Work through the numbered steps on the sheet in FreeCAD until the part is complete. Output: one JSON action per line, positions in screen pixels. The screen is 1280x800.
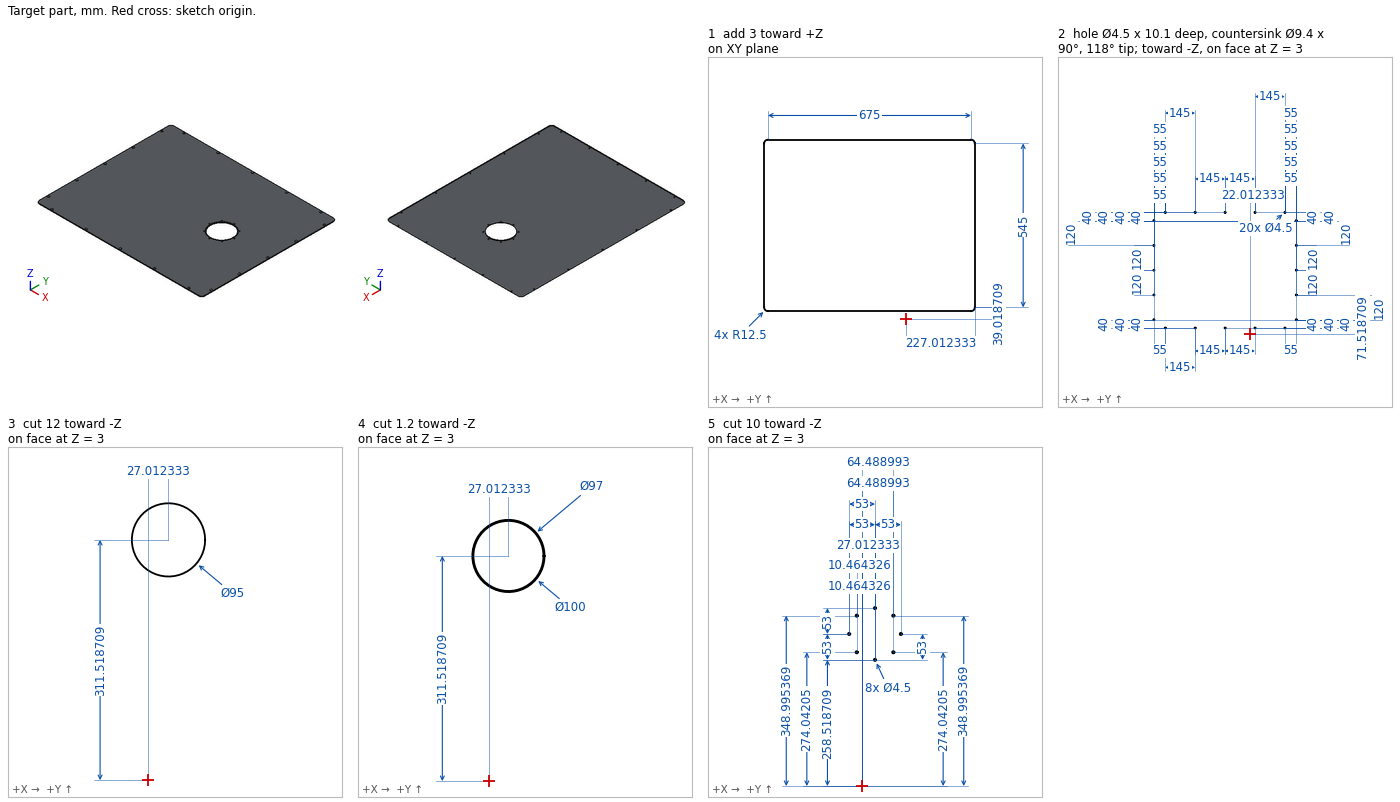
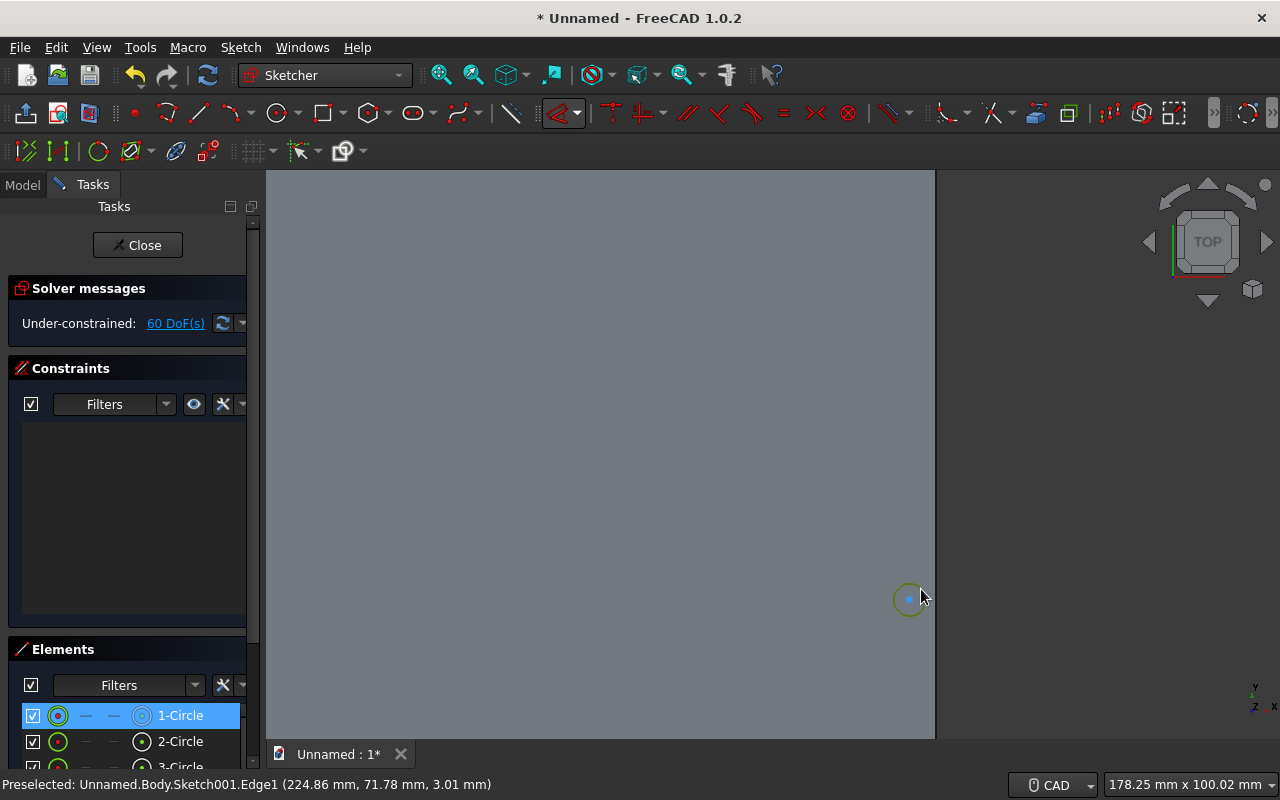
{"action": "scroll", "coordinate": [924, 597], "scroll_direction": "down", "scroll_amount": 11}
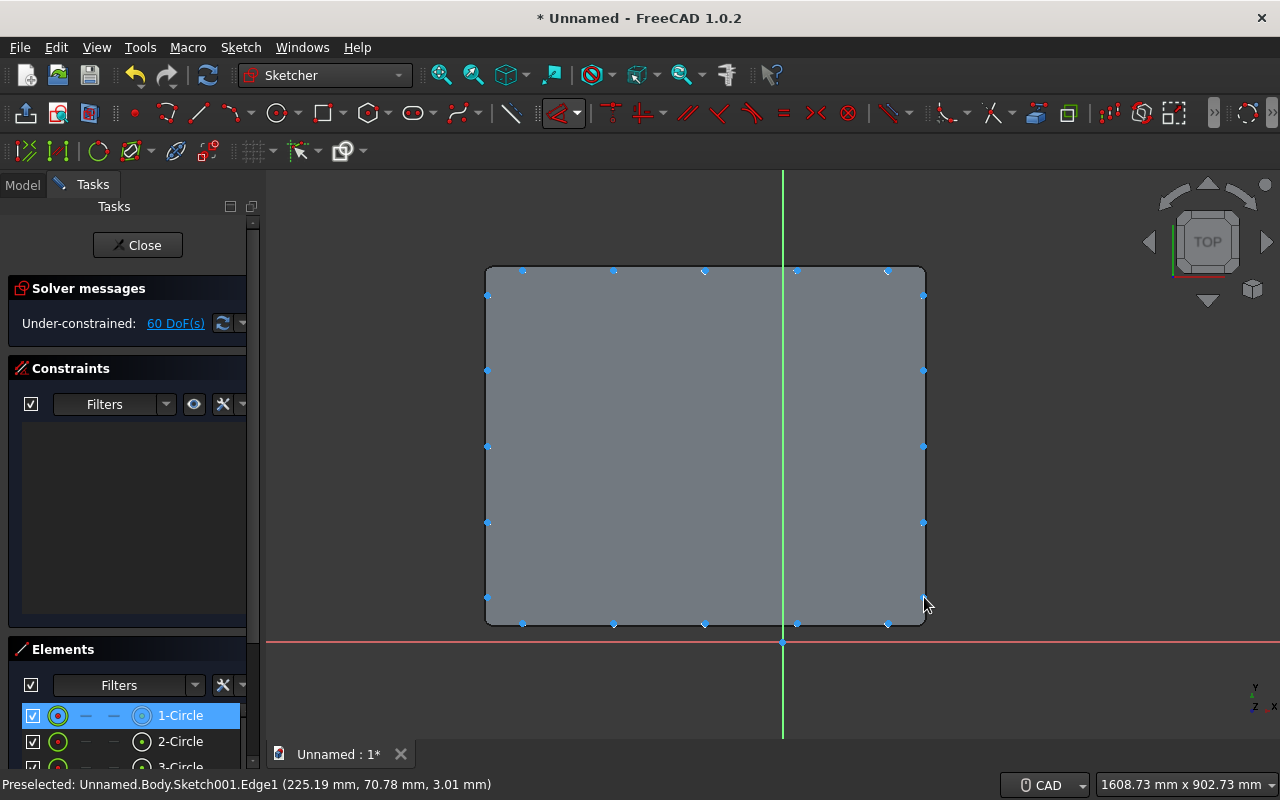
{"action": "scroll", "coordinate": [925, 521], "scroll_direction": "up", "scroll_amount": 9}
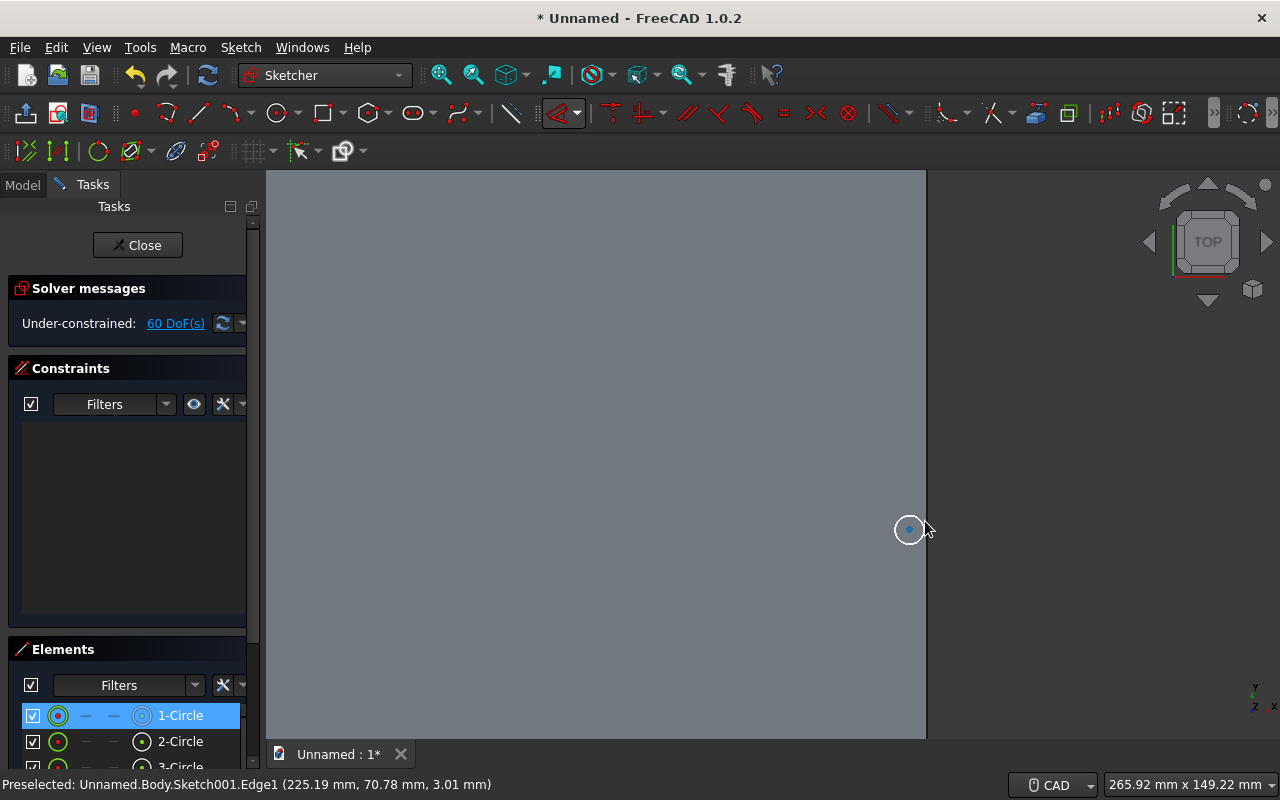
{"action": "left_click", "coordinate": [920, 520]}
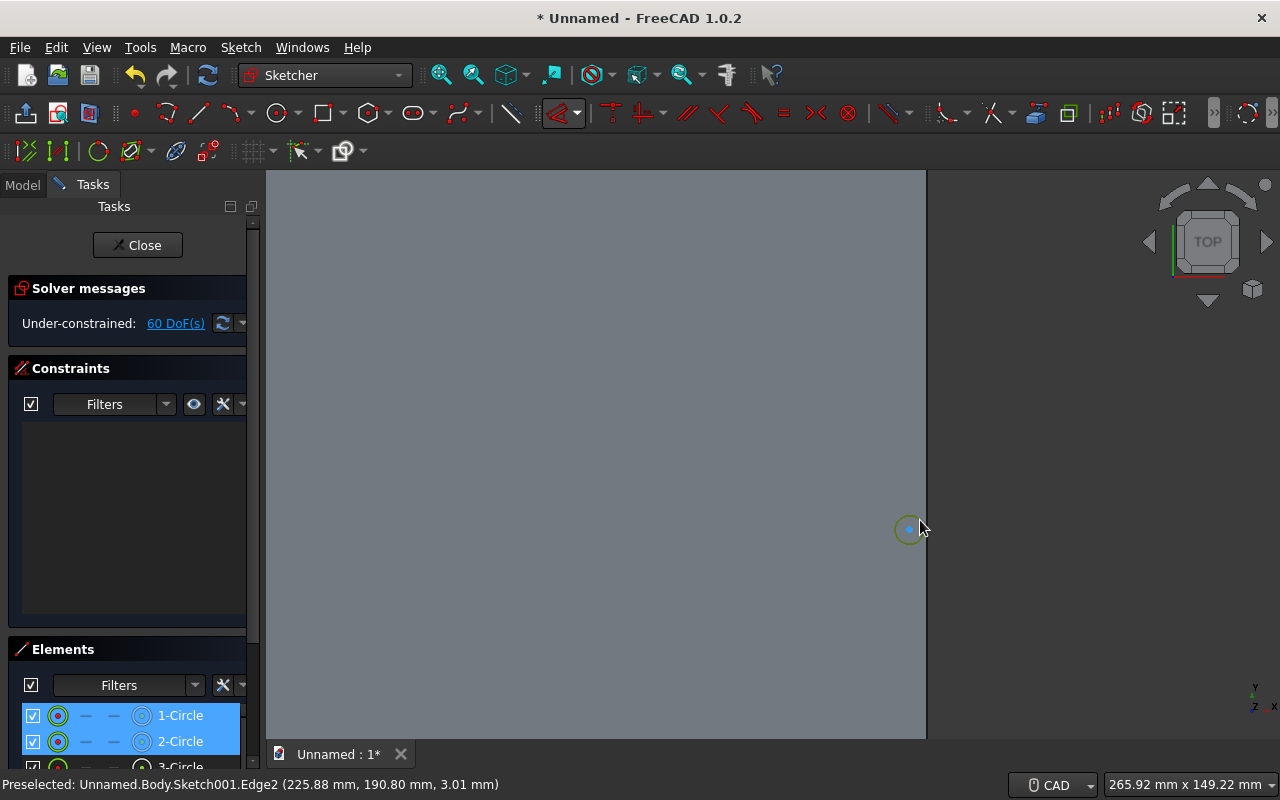
{"action": "scroll", "coordinate": [925, 521], "scroll_direction": "down", "scroll_amount": 9}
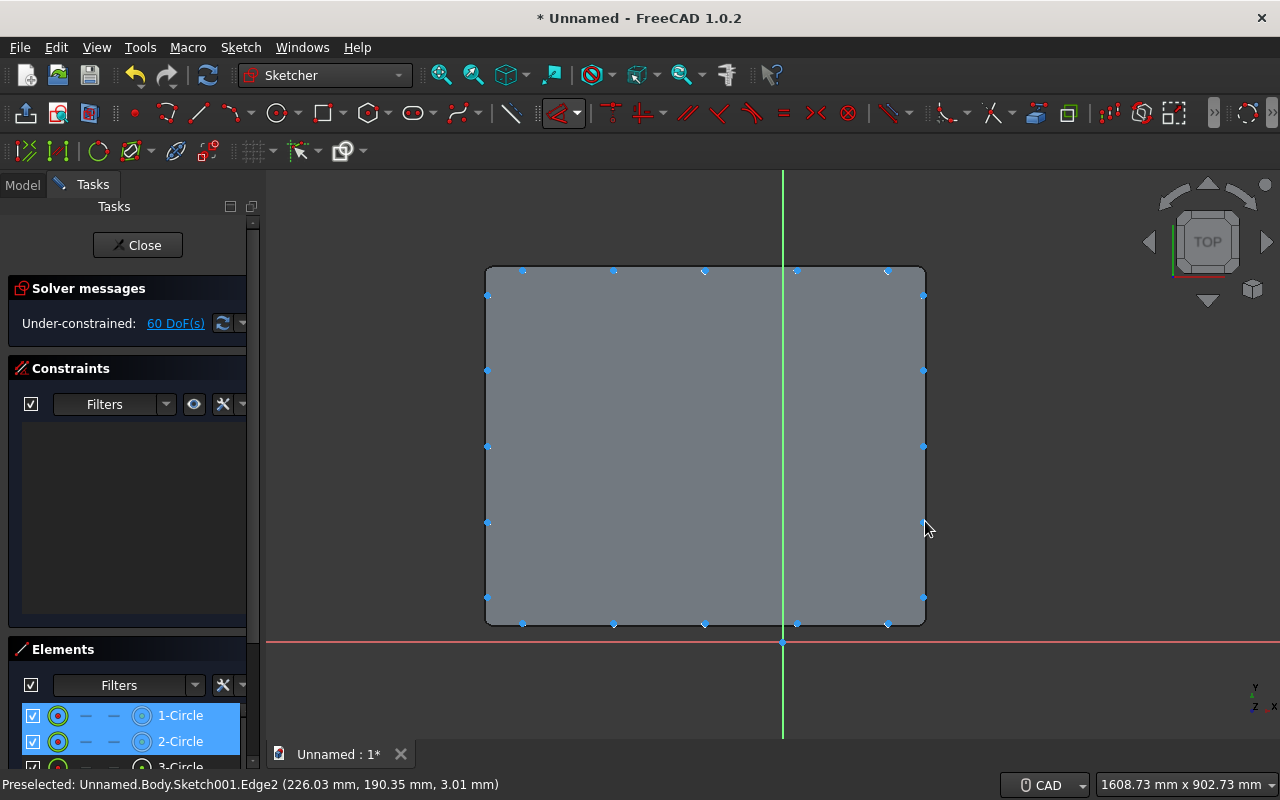
{"action": "scroll", "coordinate": [924, 446], "scroll_direction": "up", "scroll_amount": 10}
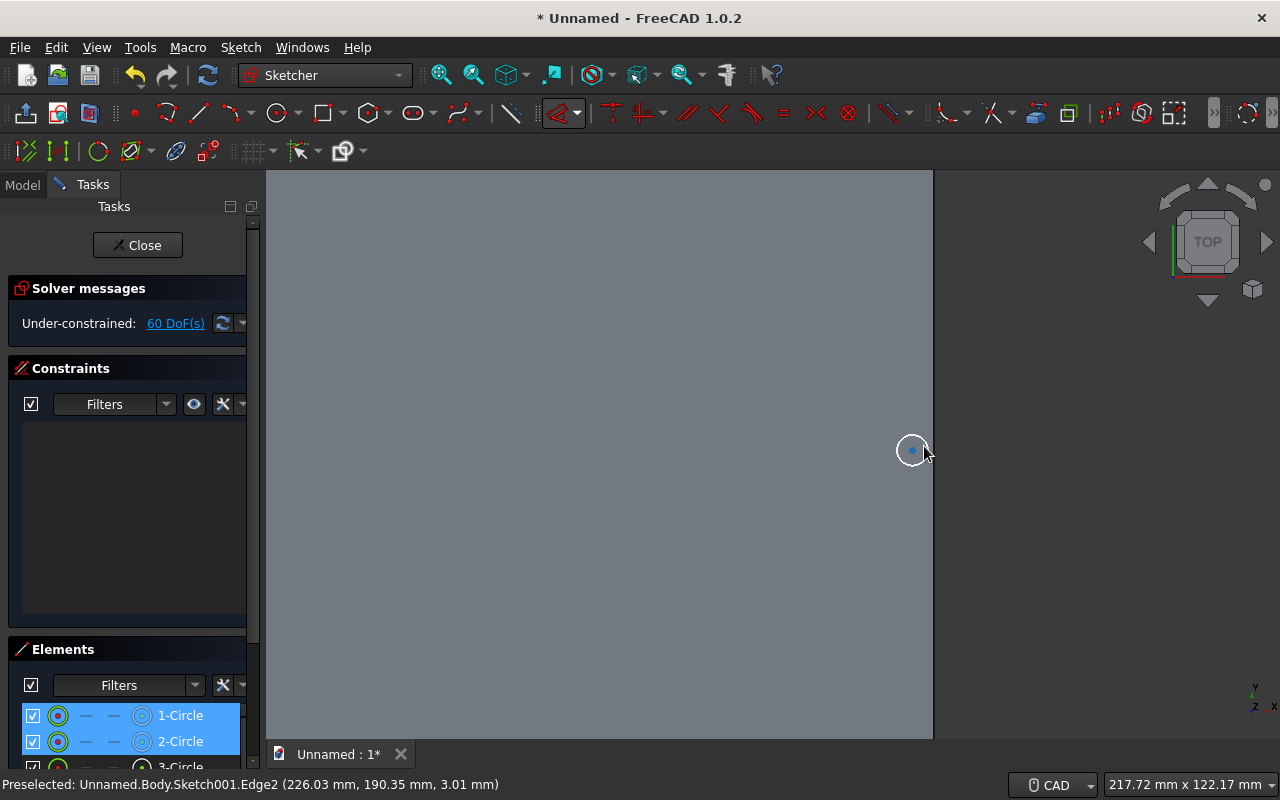
{"action": "left_click", "coordinate": [923, 439]}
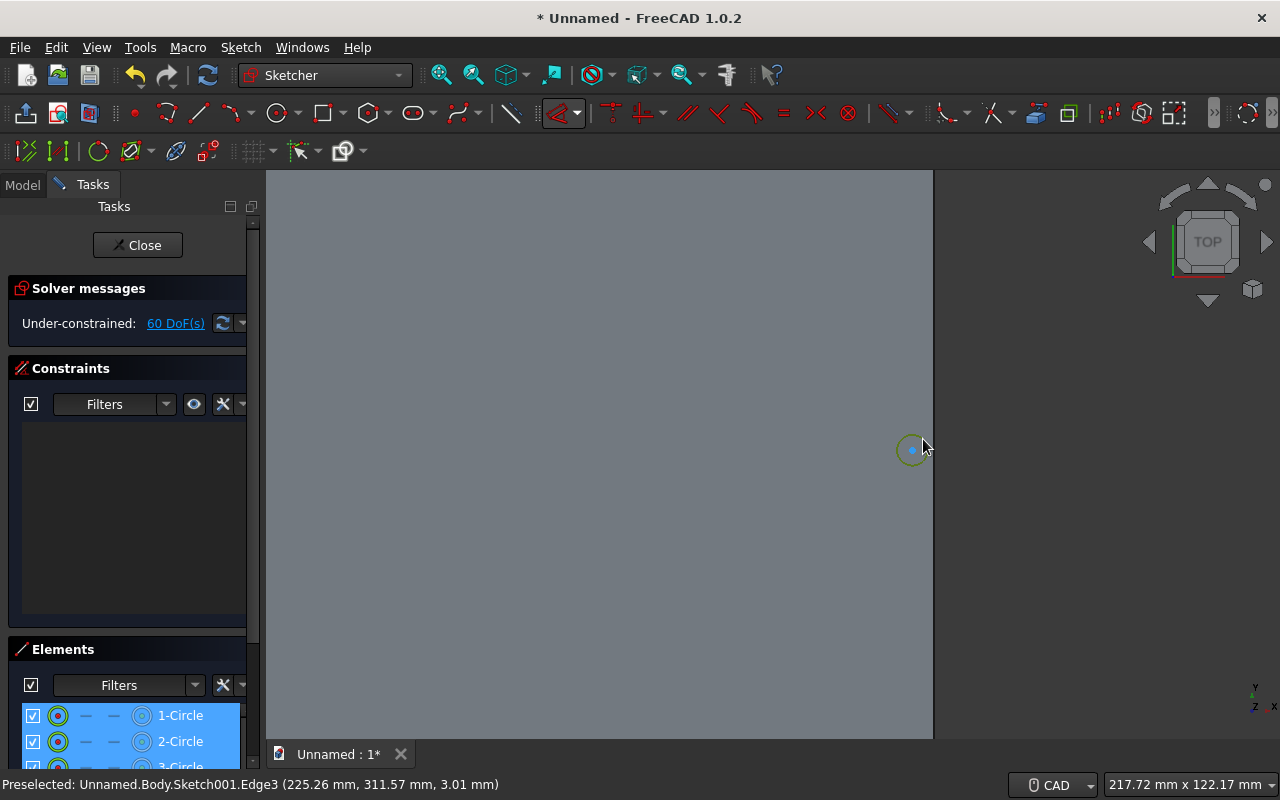
{"action": "scroll", "coordinate": [924, 446], "scroll_direction": "down", "scroll_amount": 10}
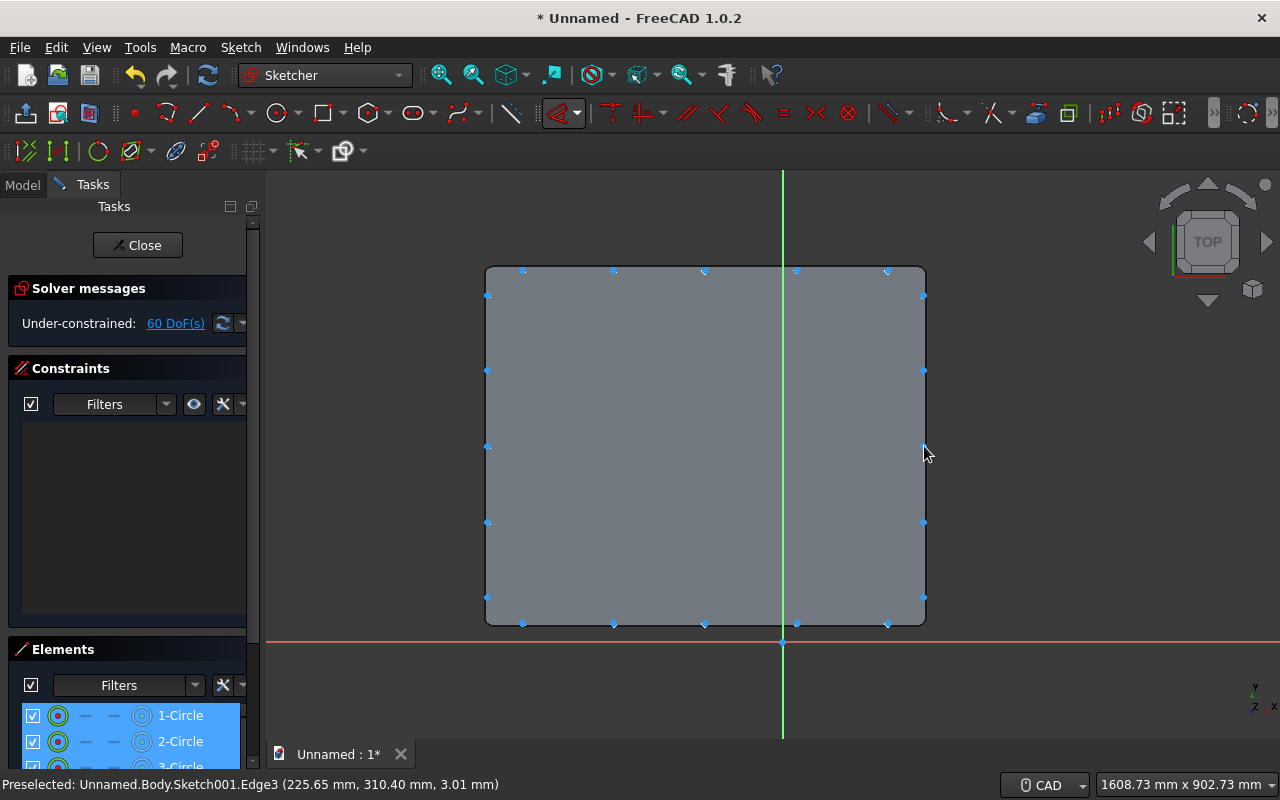
{"action": "scroll", "coordinate": [924, 370], "scroll_direction": "up", "scroll_amount": 11}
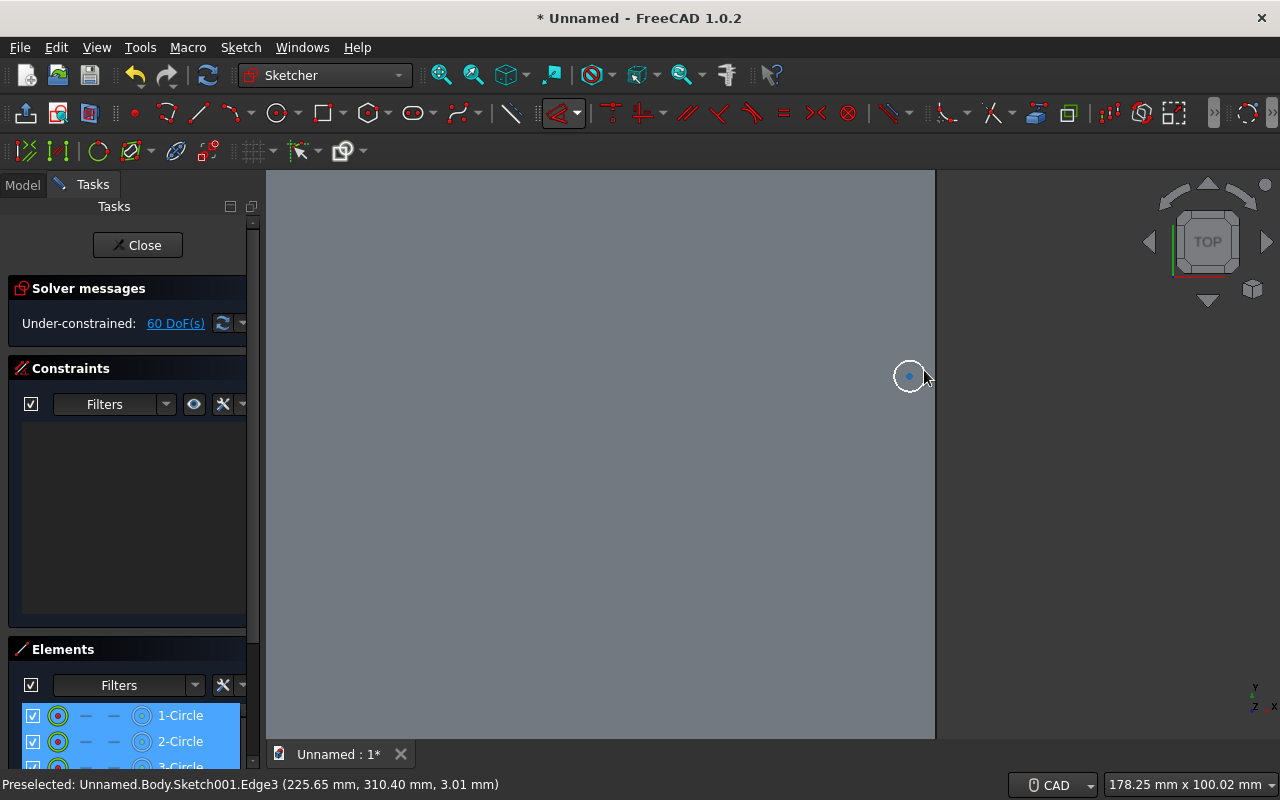
{"action": "left_click", "coordinate": [921, 365]}